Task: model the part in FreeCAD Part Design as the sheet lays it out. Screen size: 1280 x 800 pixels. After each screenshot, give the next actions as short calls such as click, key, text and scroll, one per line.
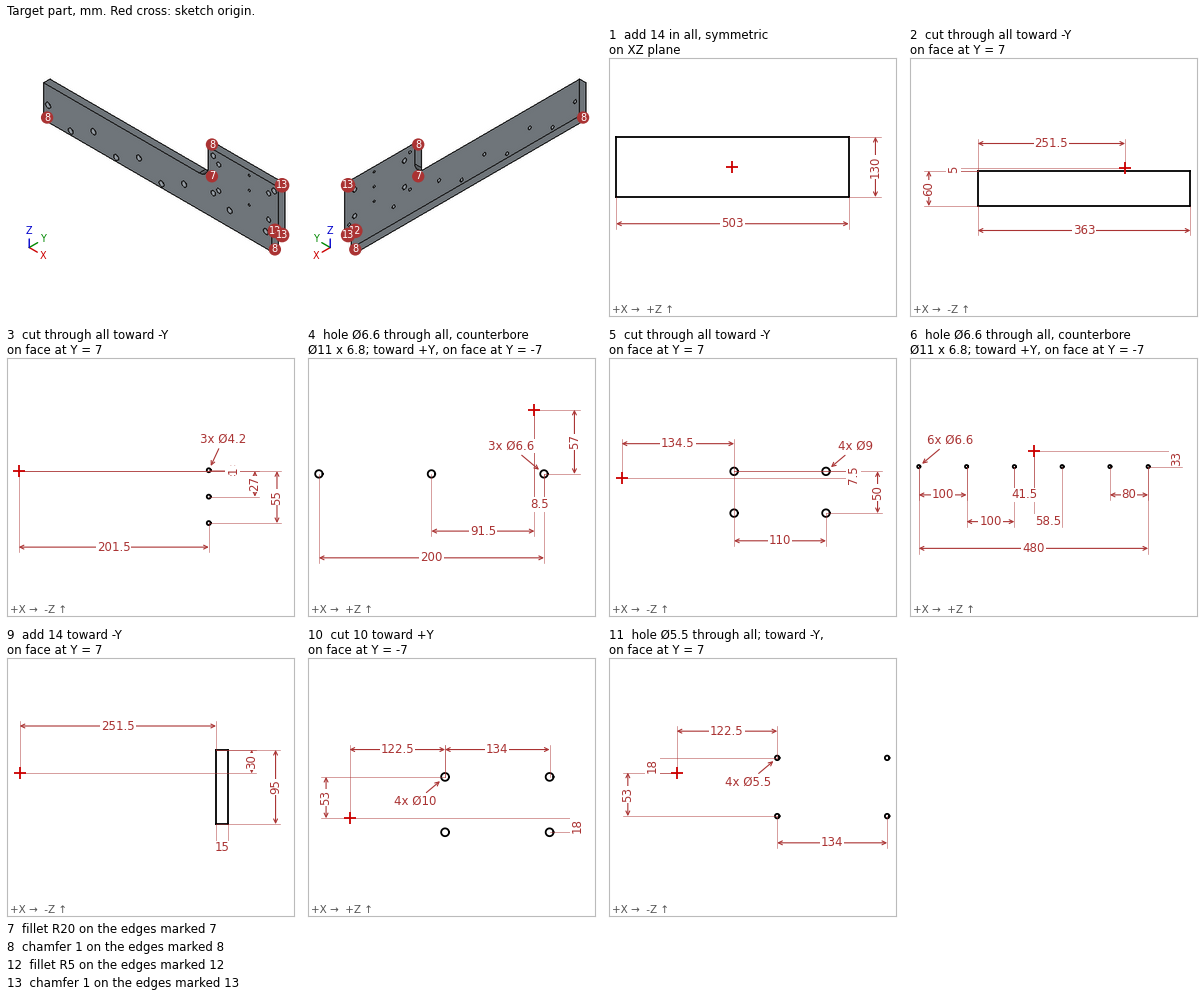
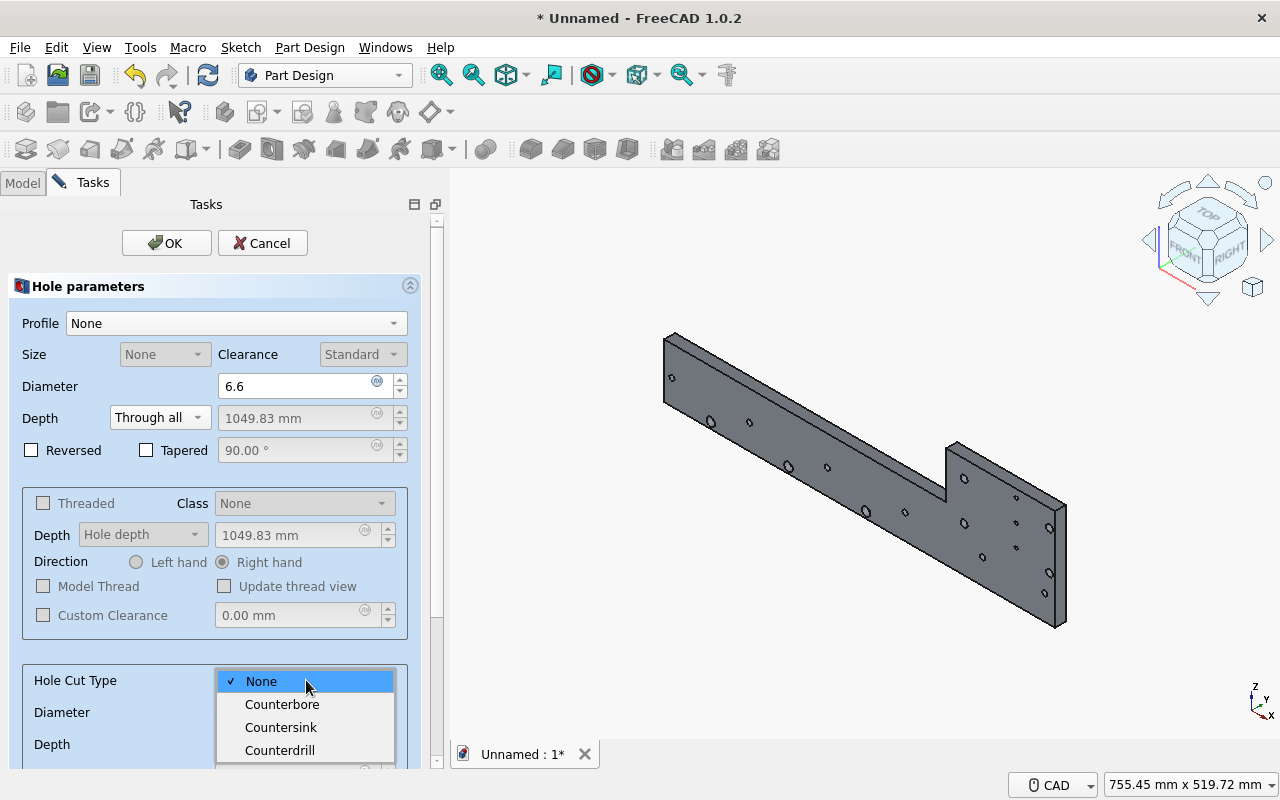
click(304, 704)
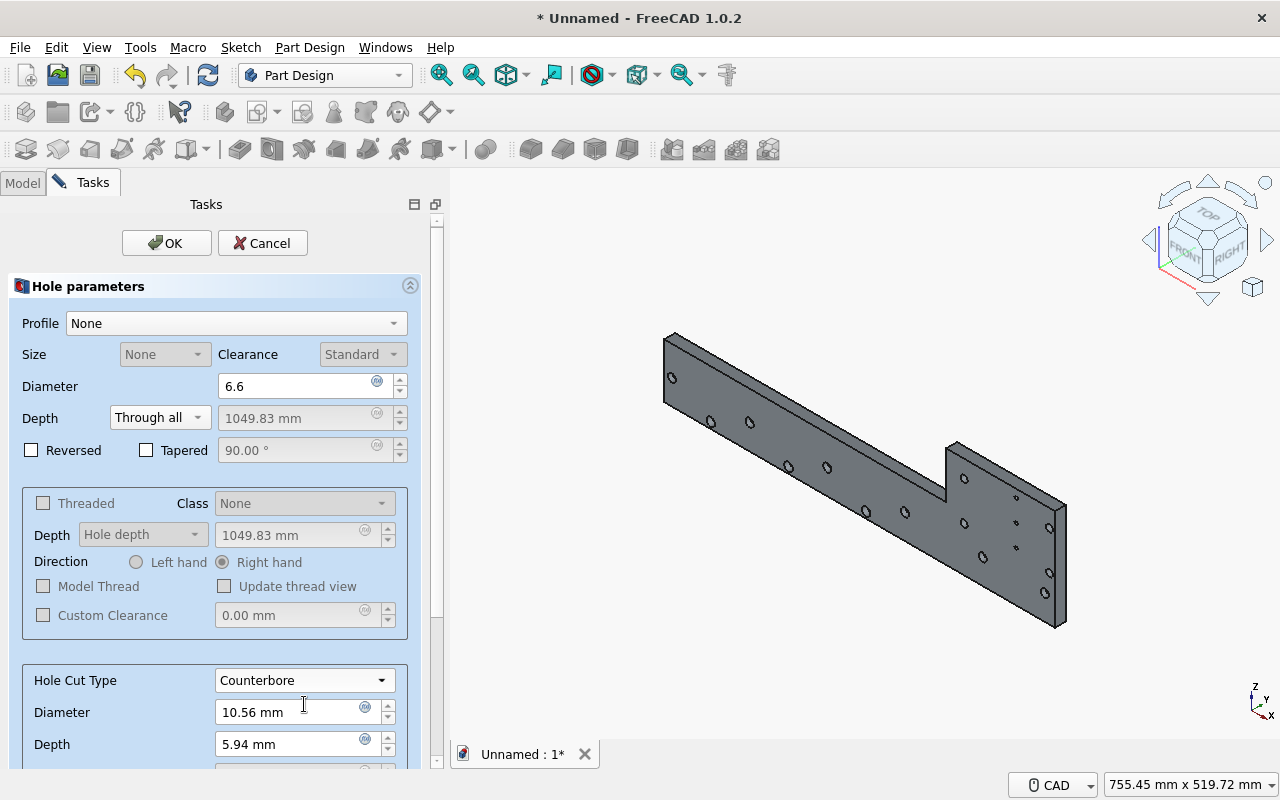
triple_click(298, 712)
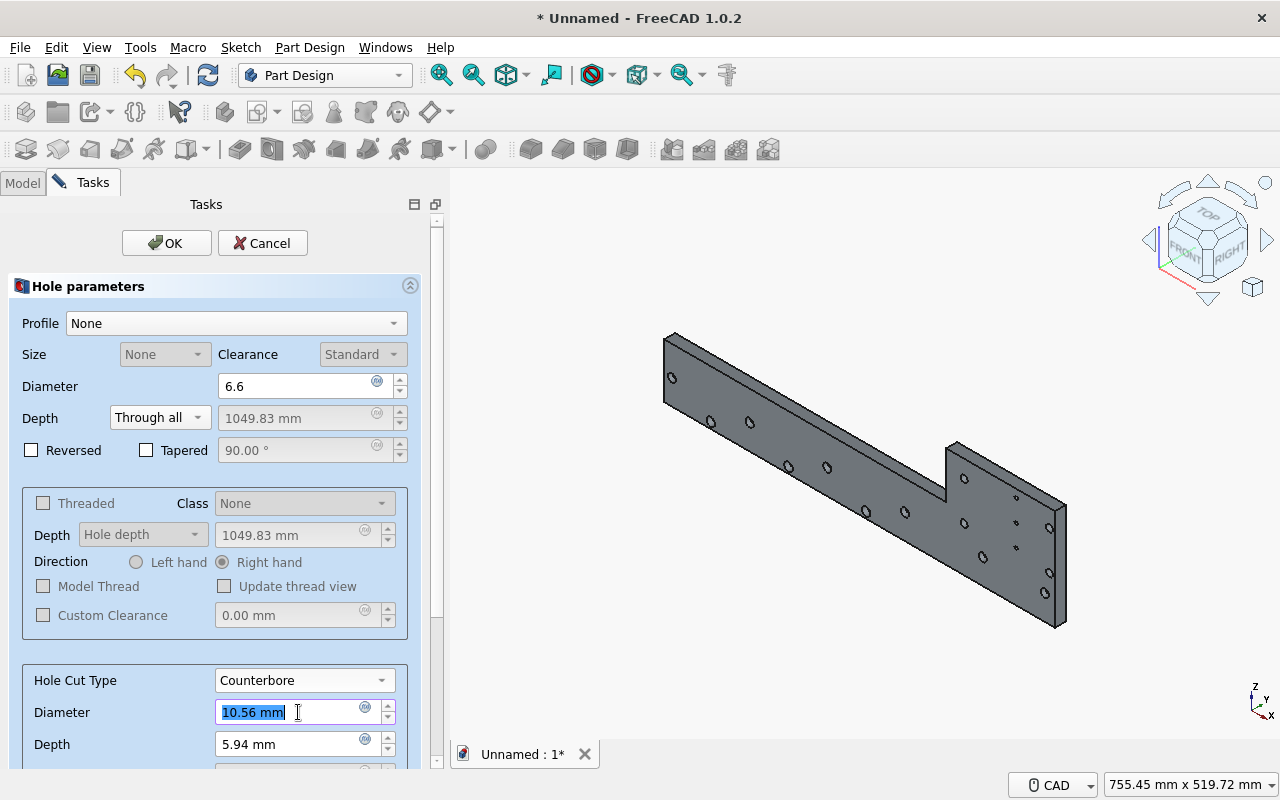
text(11)
key(Tab)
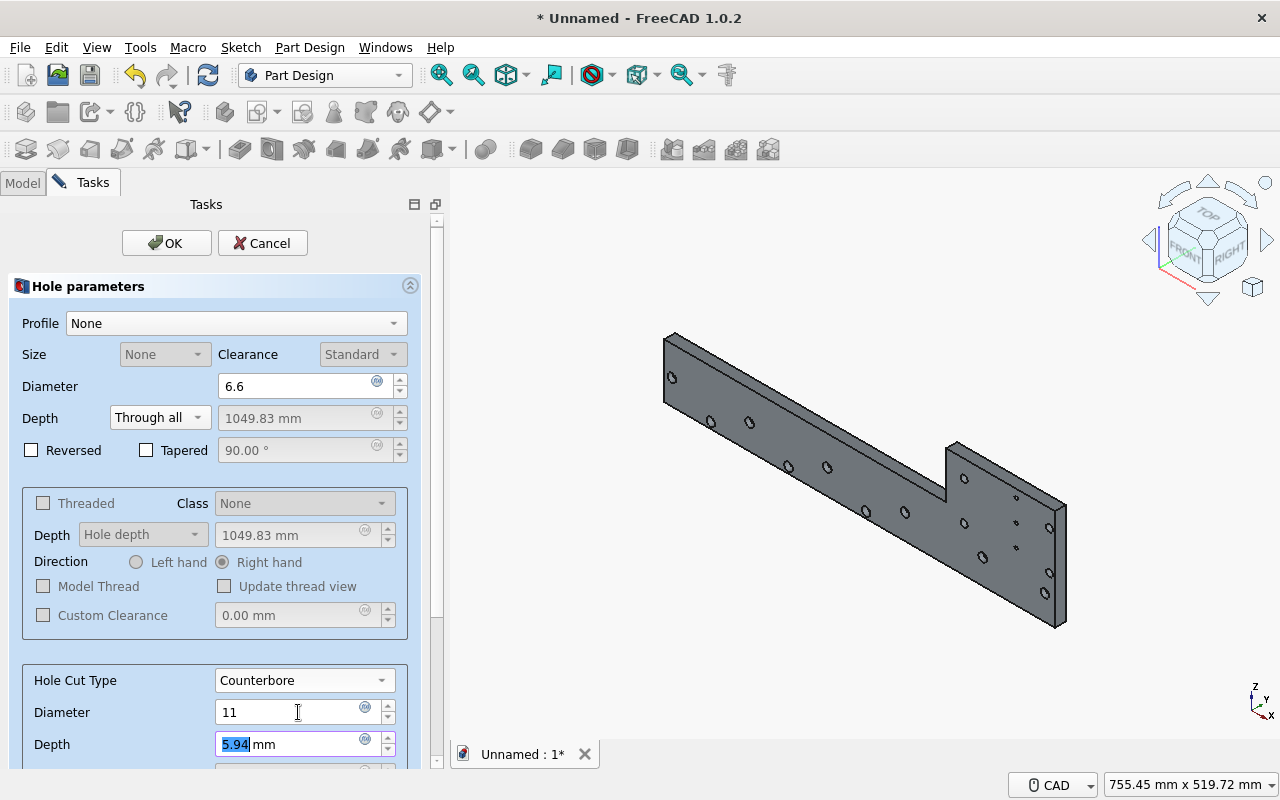
text(6.8)
key(Tab)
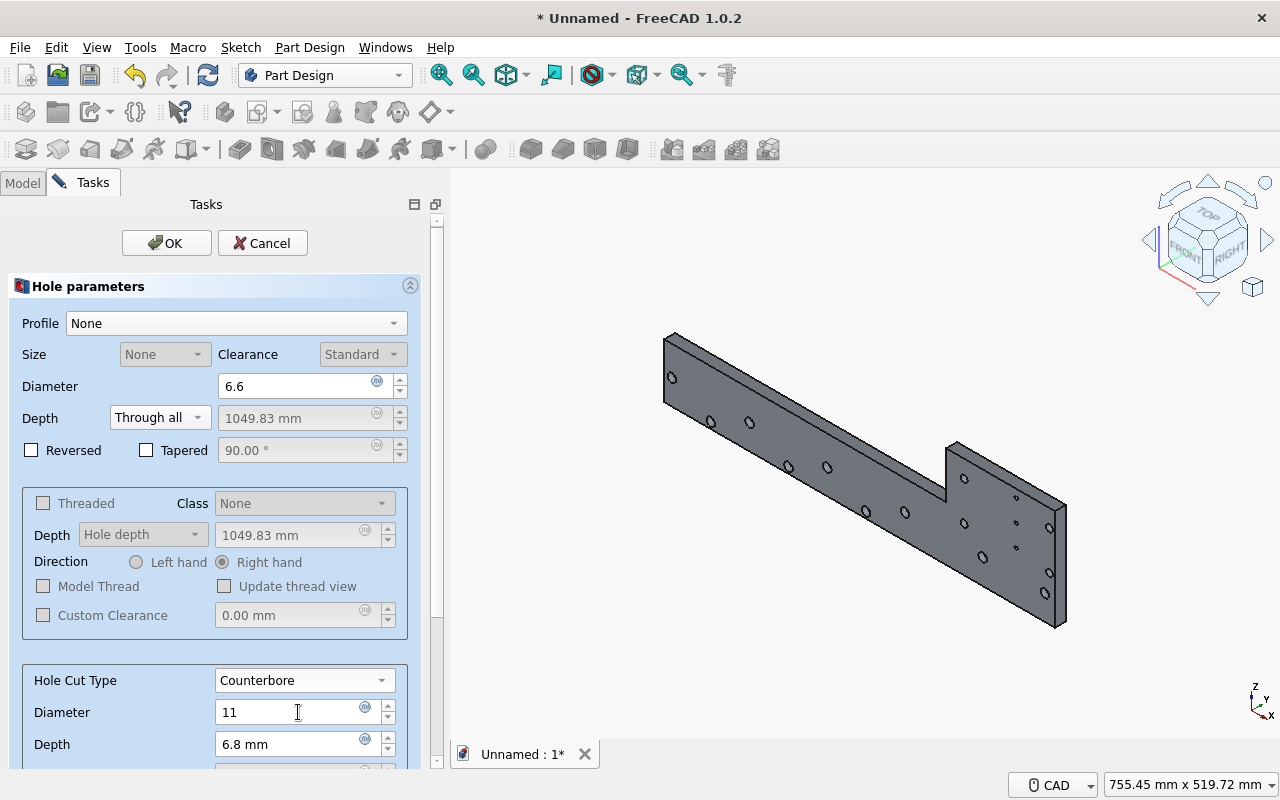
click(167, 243)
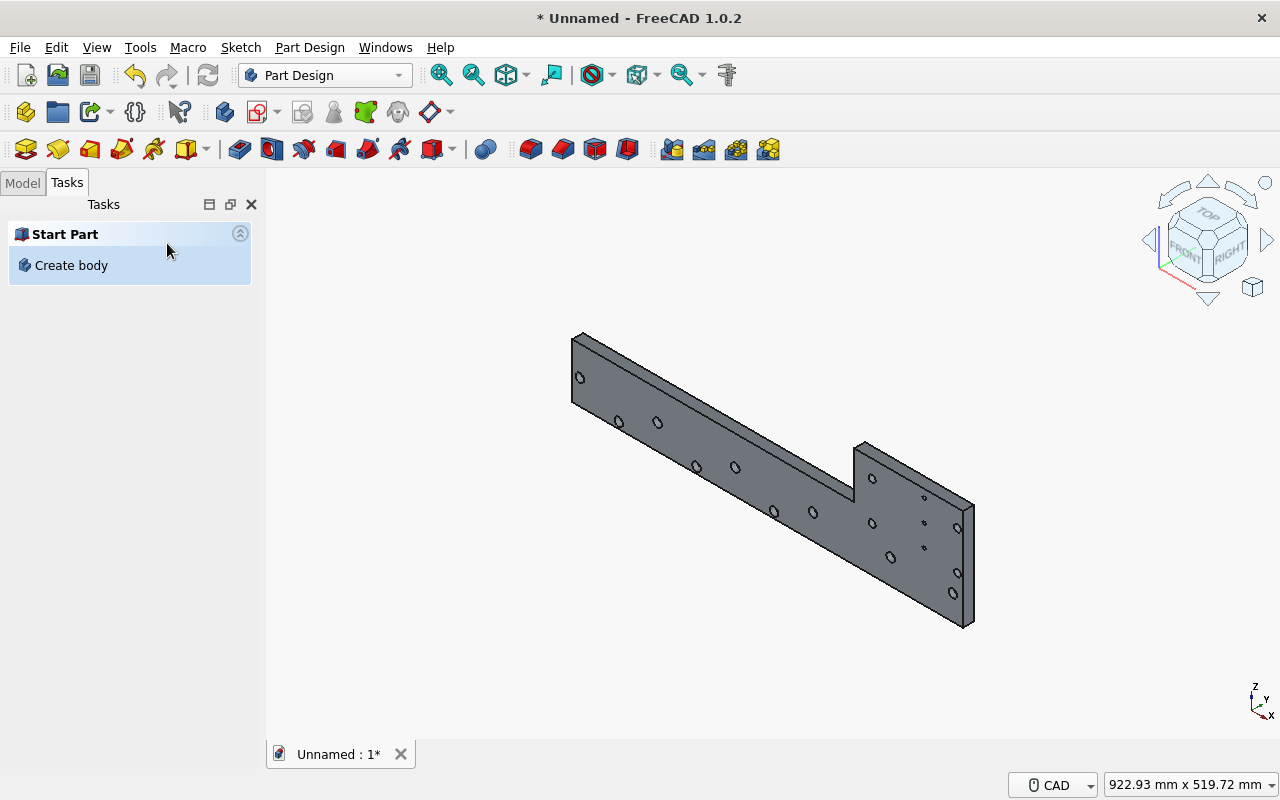
scroll(860, 498, up, 5)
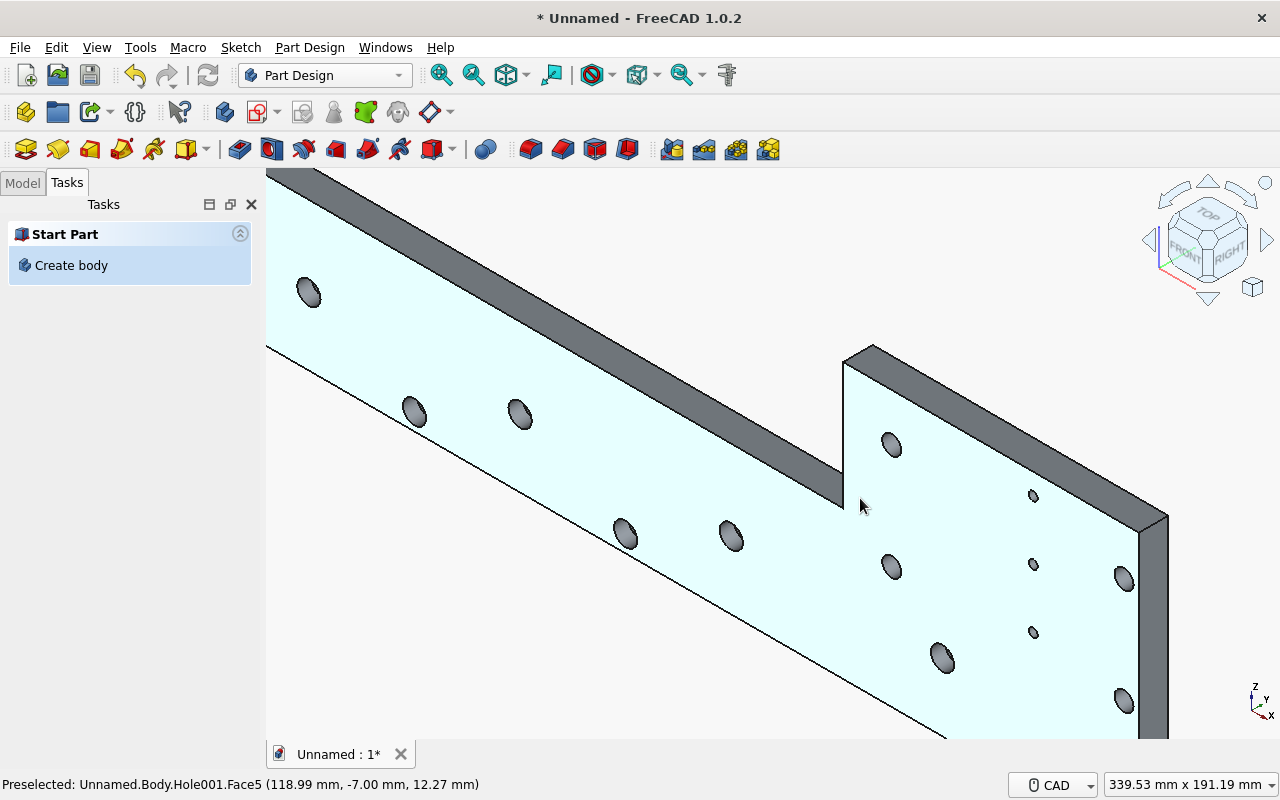
key(v)
key(f)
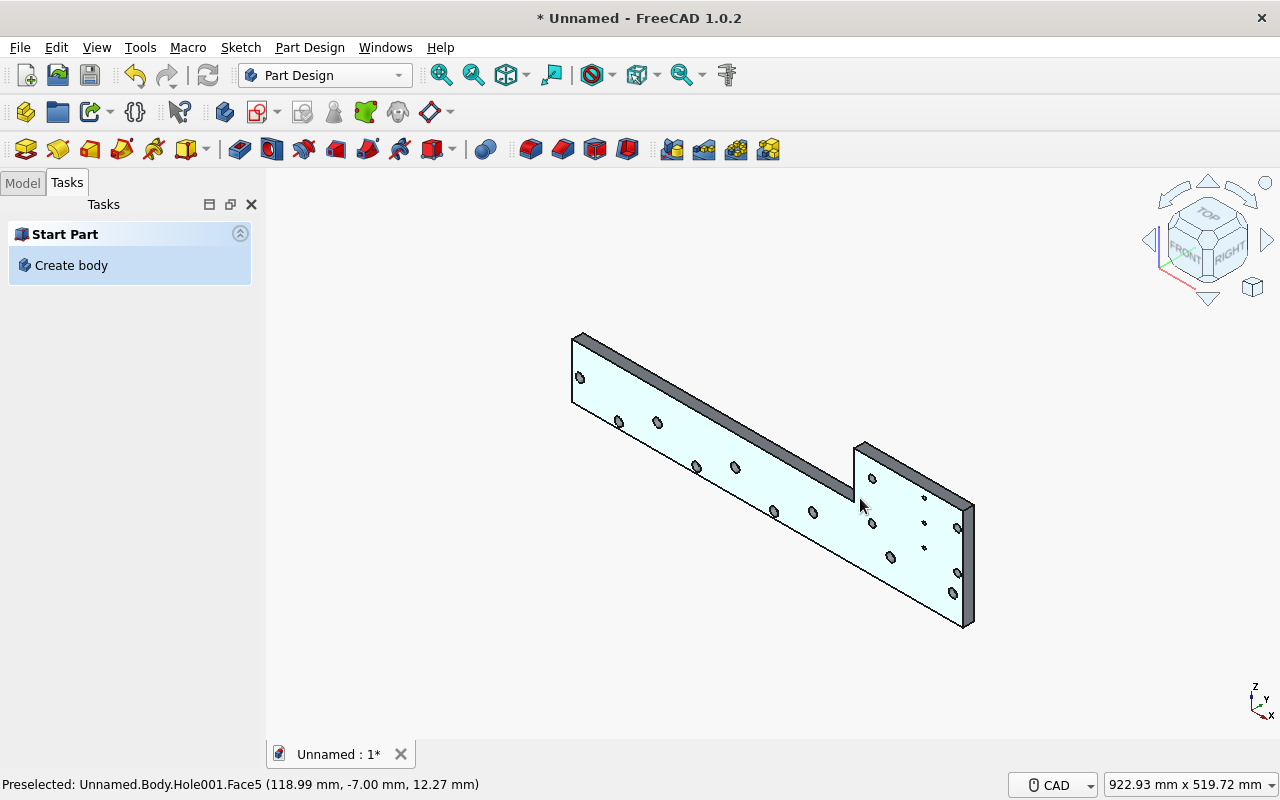
key(2)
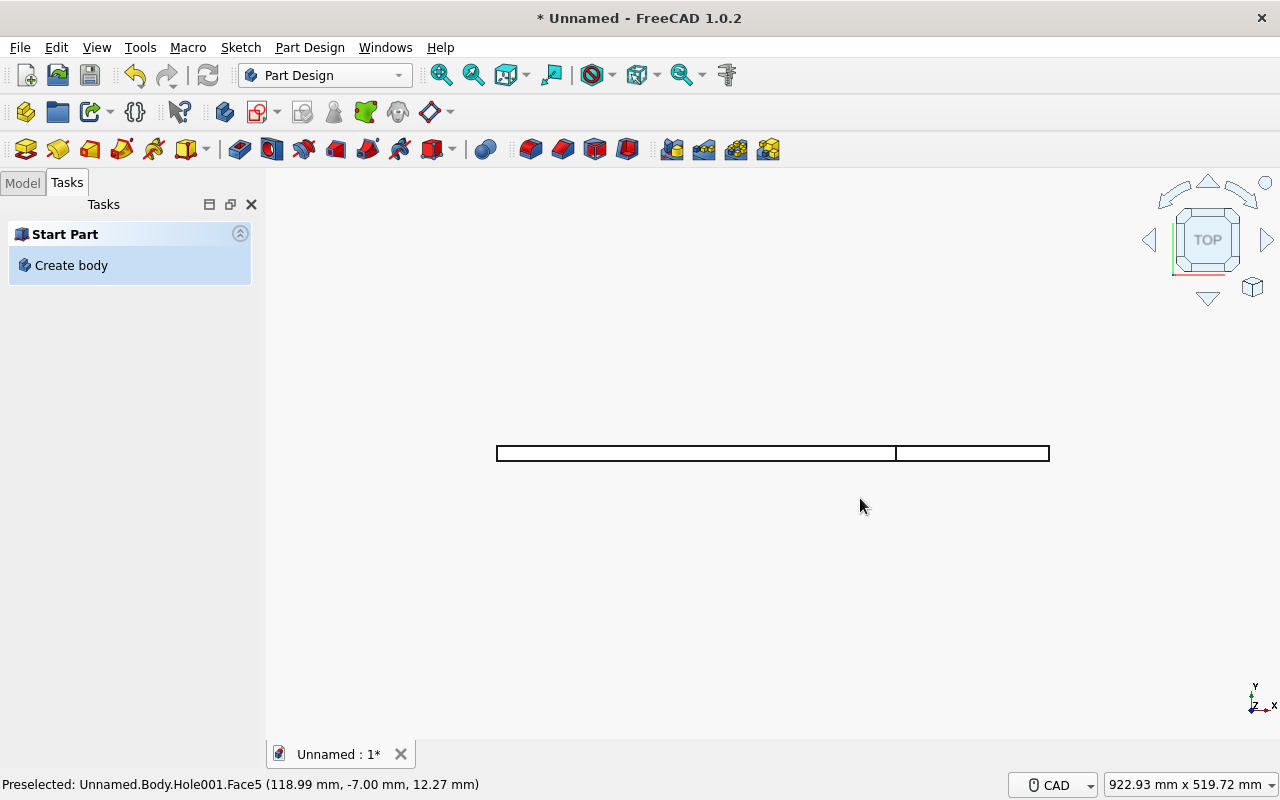
scroll(896, 452, up, 5)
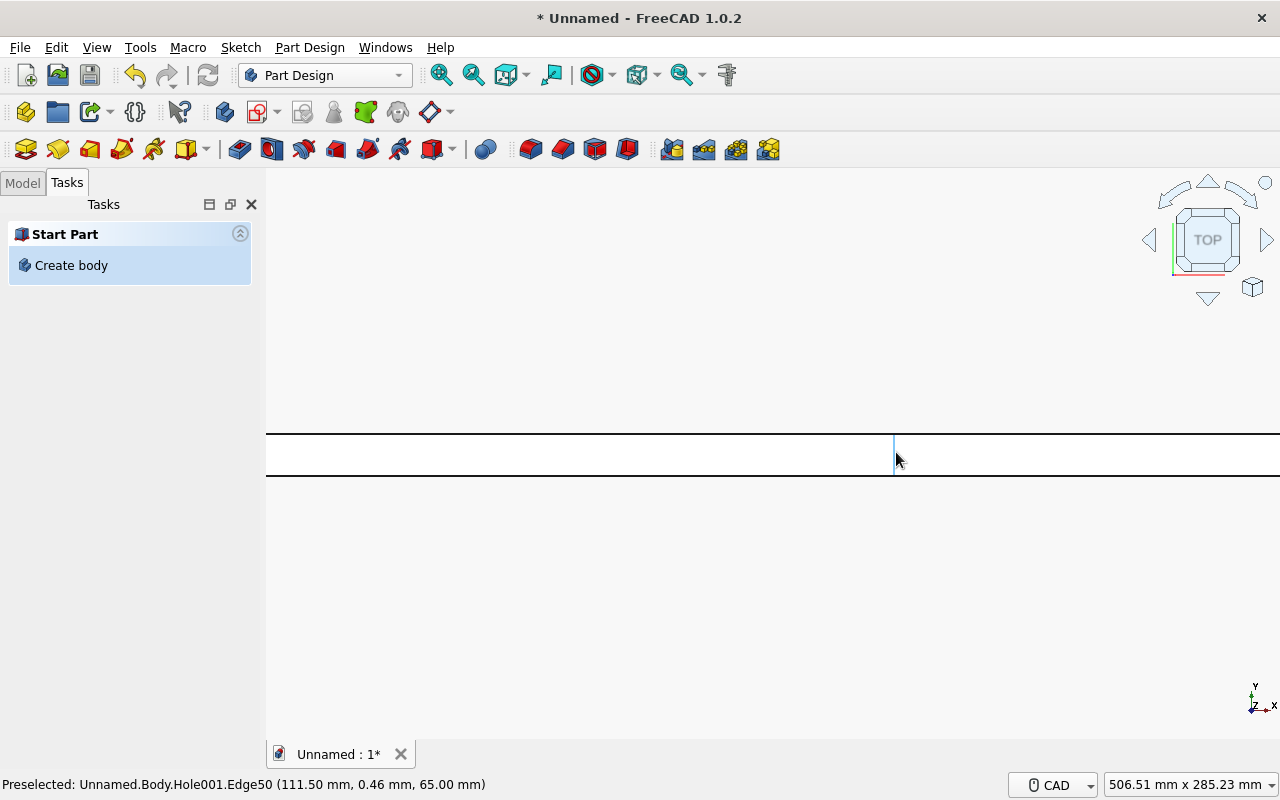
key(v)
key(f)